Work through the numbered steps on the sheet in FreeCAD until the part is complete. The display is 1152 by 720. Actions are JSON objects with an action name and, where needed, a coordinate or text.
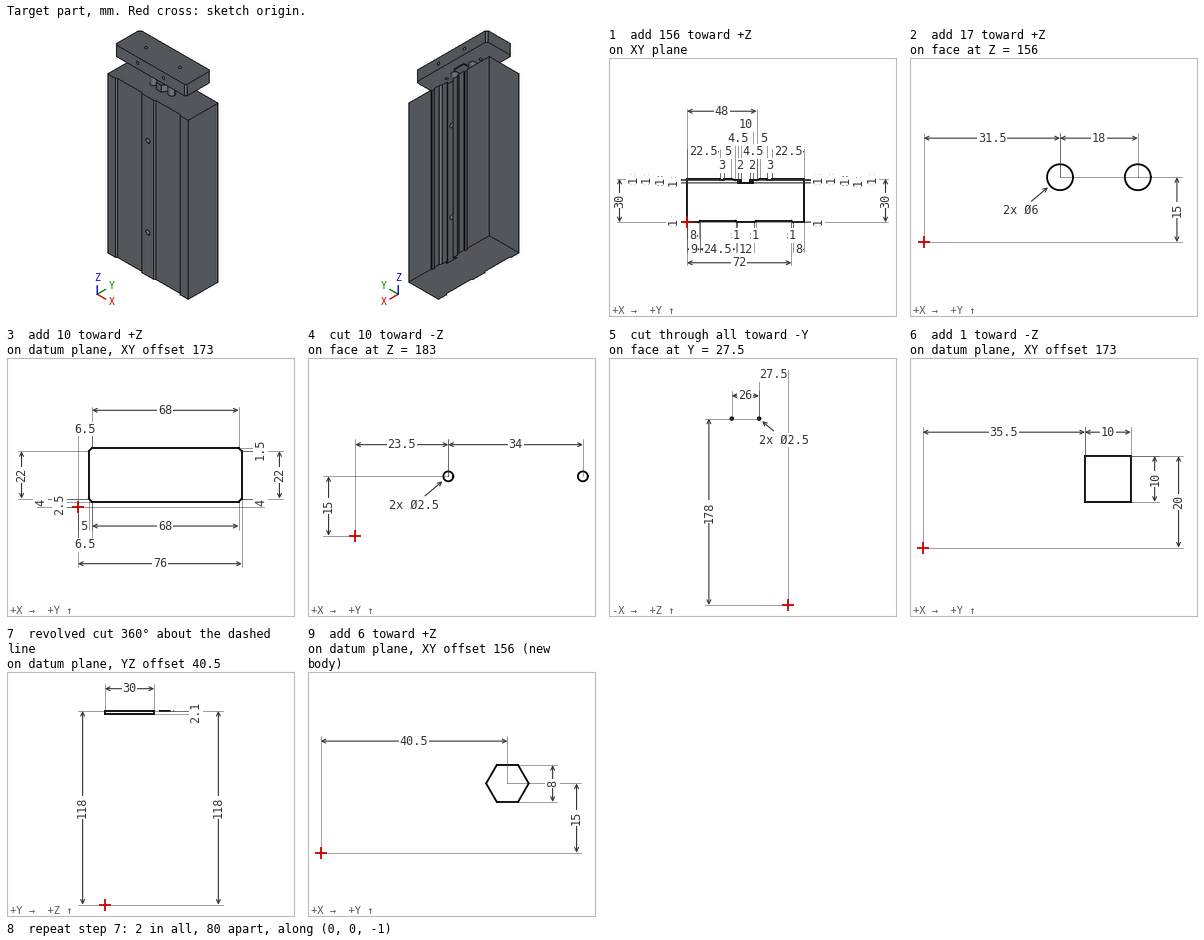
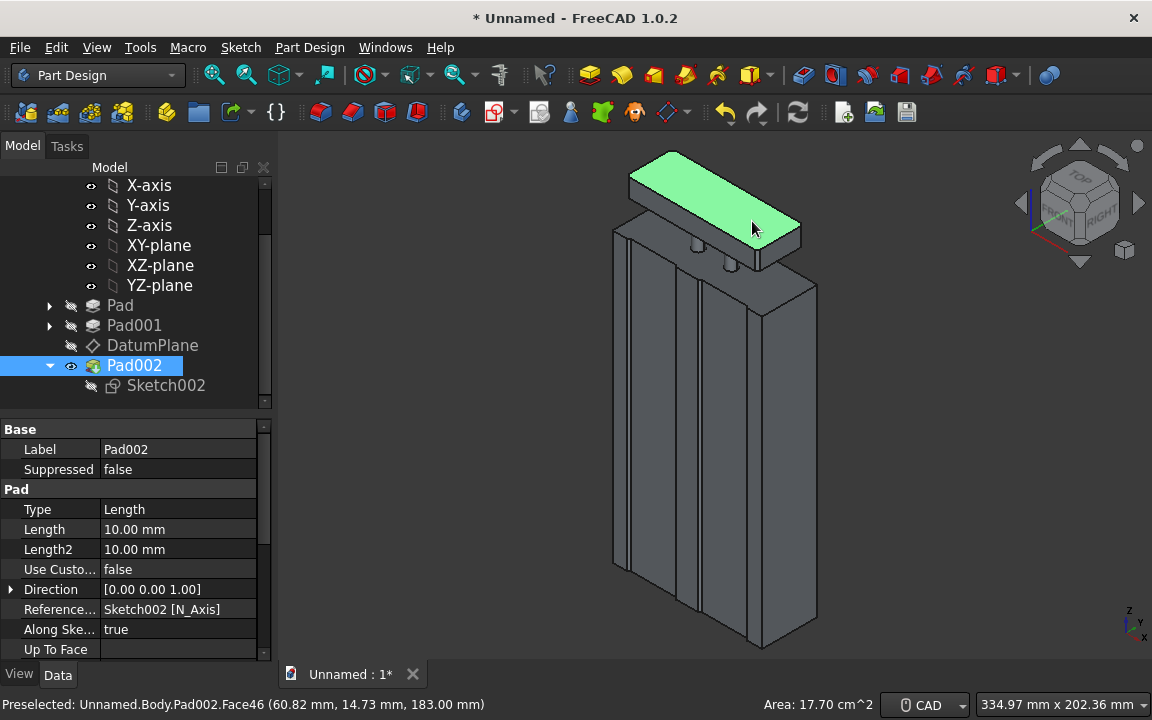
{"action": "left_click", "coordinate": [494, 112]}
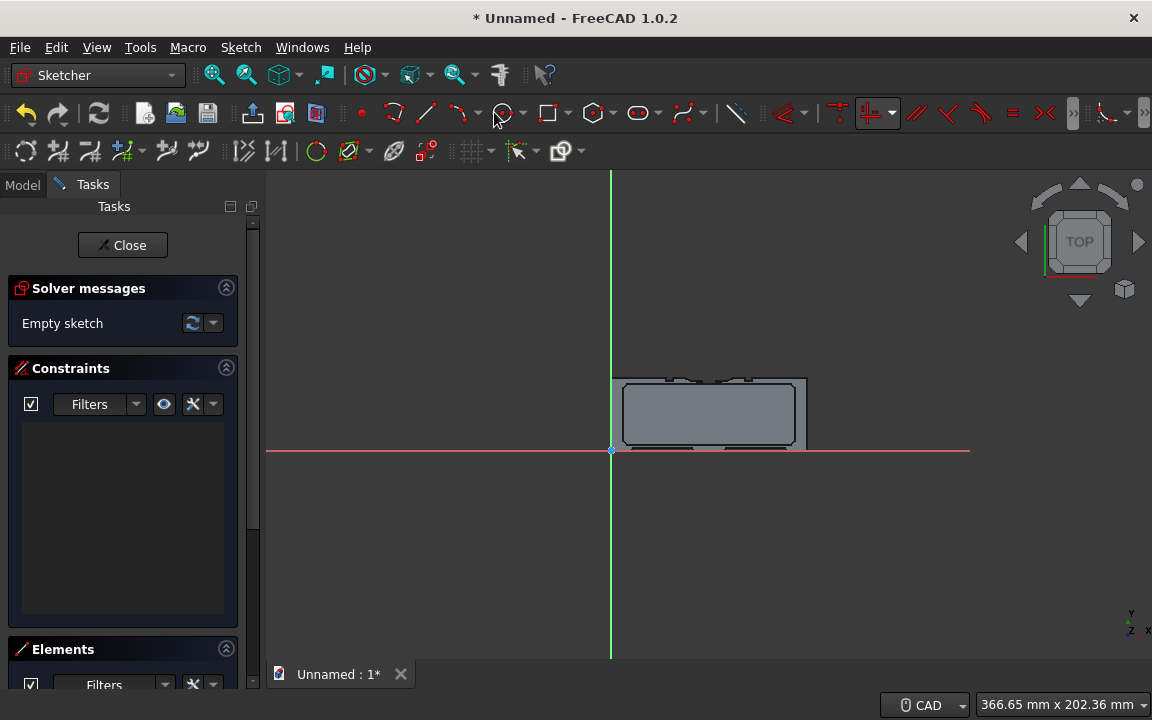
{"action": "scroll", "coordinate": [700, 438], "scroll_direction": "up", "scroll_amount": 6}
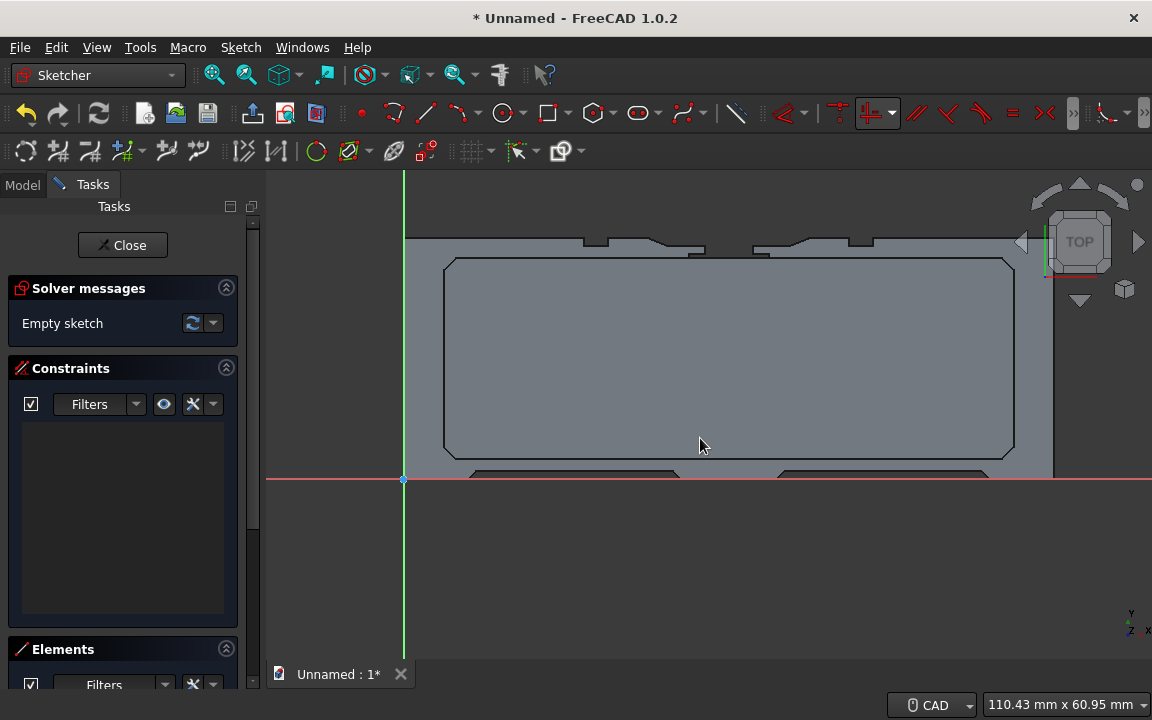
{"action": "left_click", "coordinate": [504, 114]}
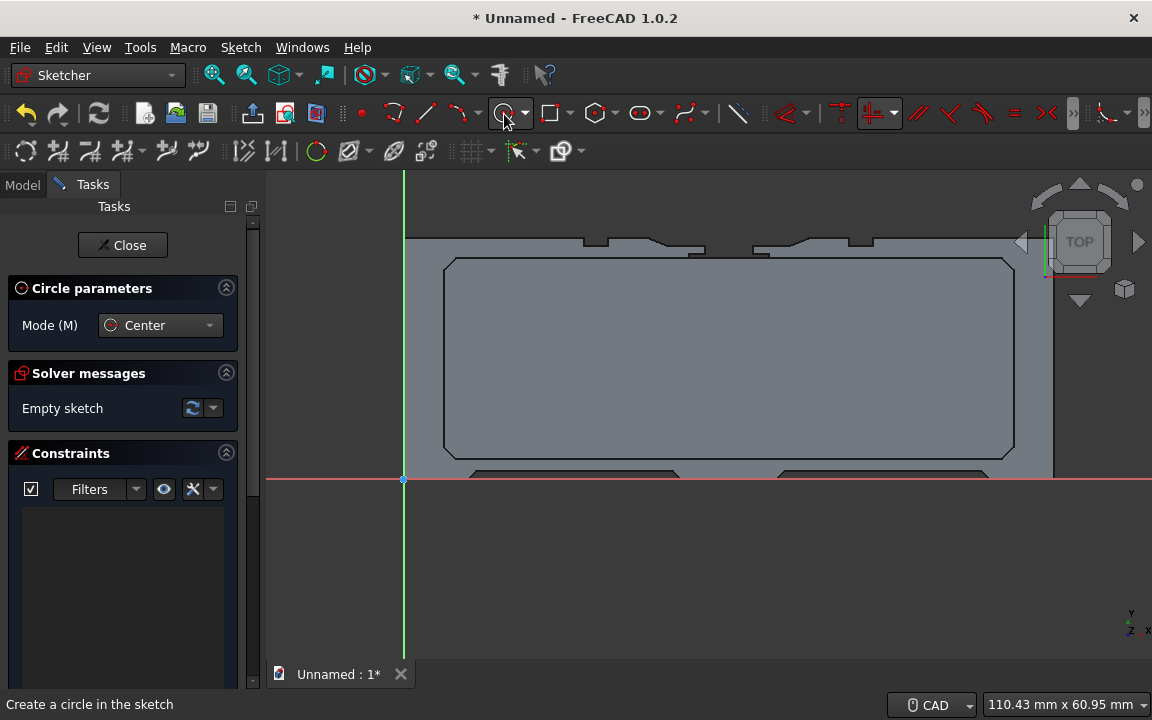
{"action": "scroll", "coordinate": [592, 359], "scroll_direction": "up", "scroll_amount": 5}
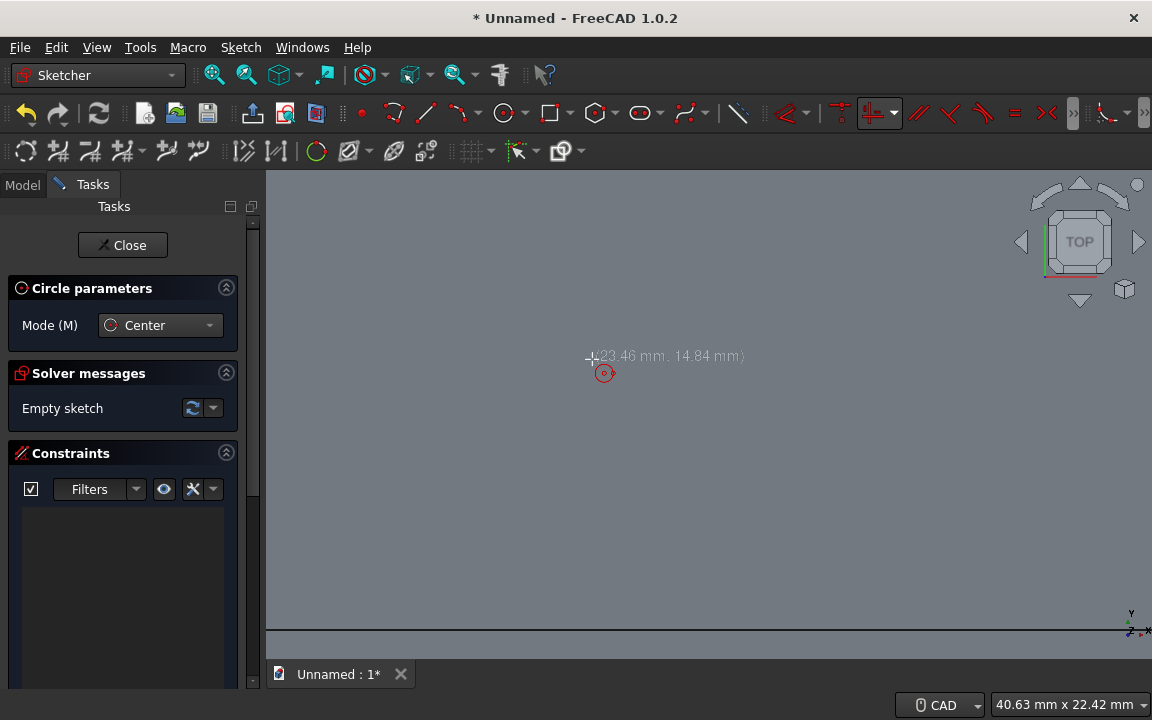
{"action": "left_click", "coordinate": [592, 358]}
{"action": "mouse_move", "coordinate": [612, 338]}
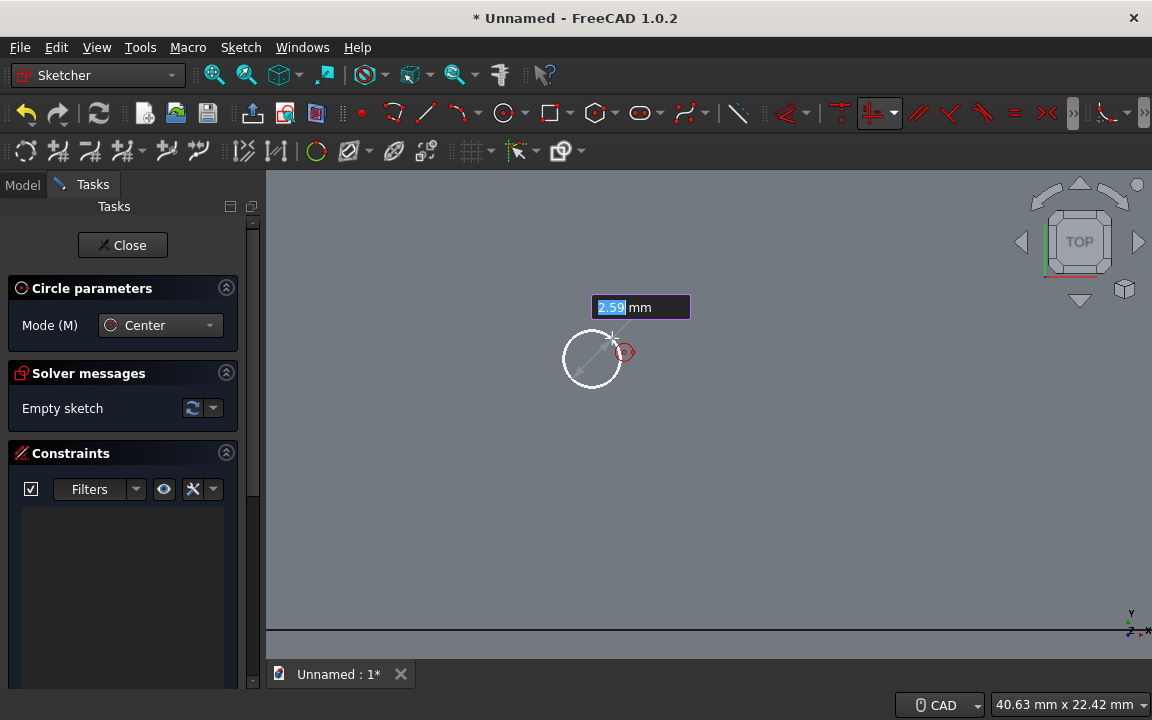
{"action": "type", "text": "2.5"}
{"action": "key", "text": "Return"}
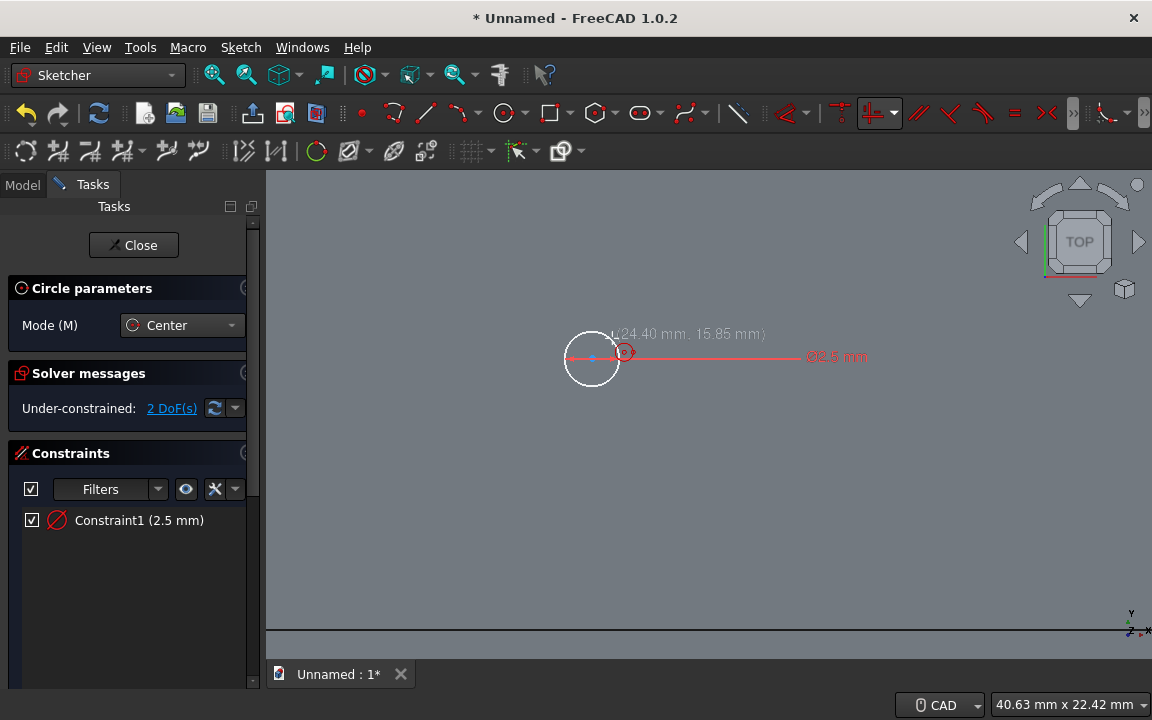
{"action": "scroll", "coordinate": [594, 360], "scroll_direction": "down", "scroll_amount": 5}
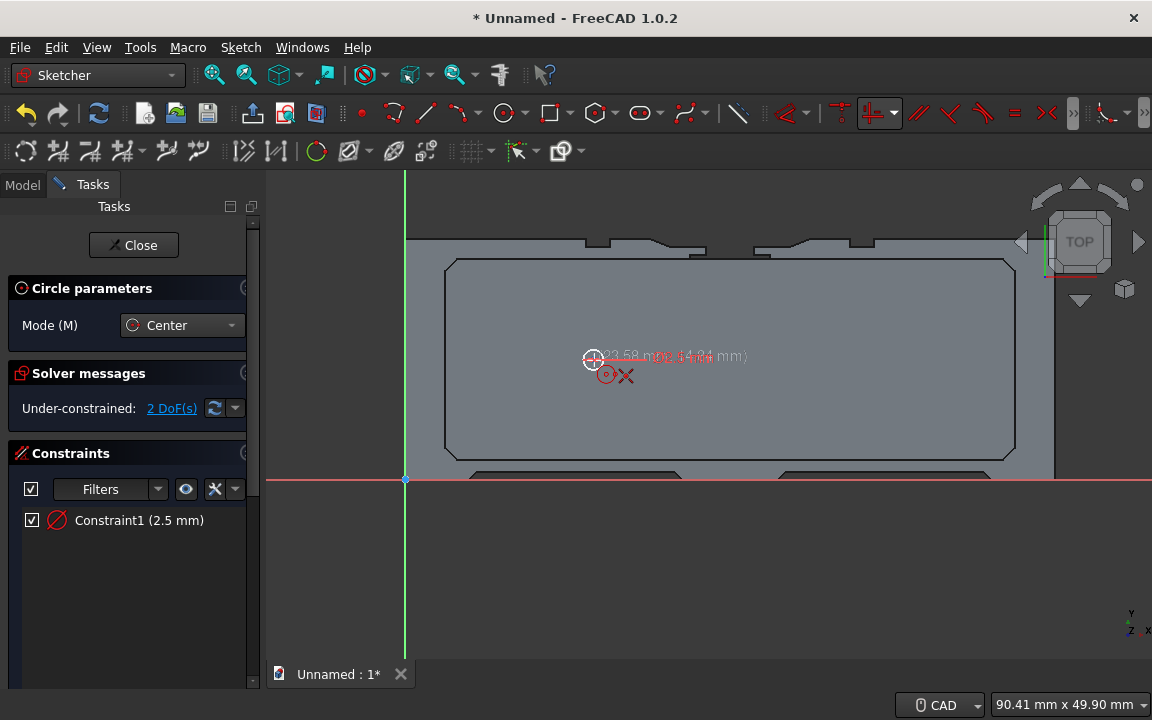
{"action": "scroll", "coordinate": [866, 359], "scroll_direction": "up", "scroll_amount": 5}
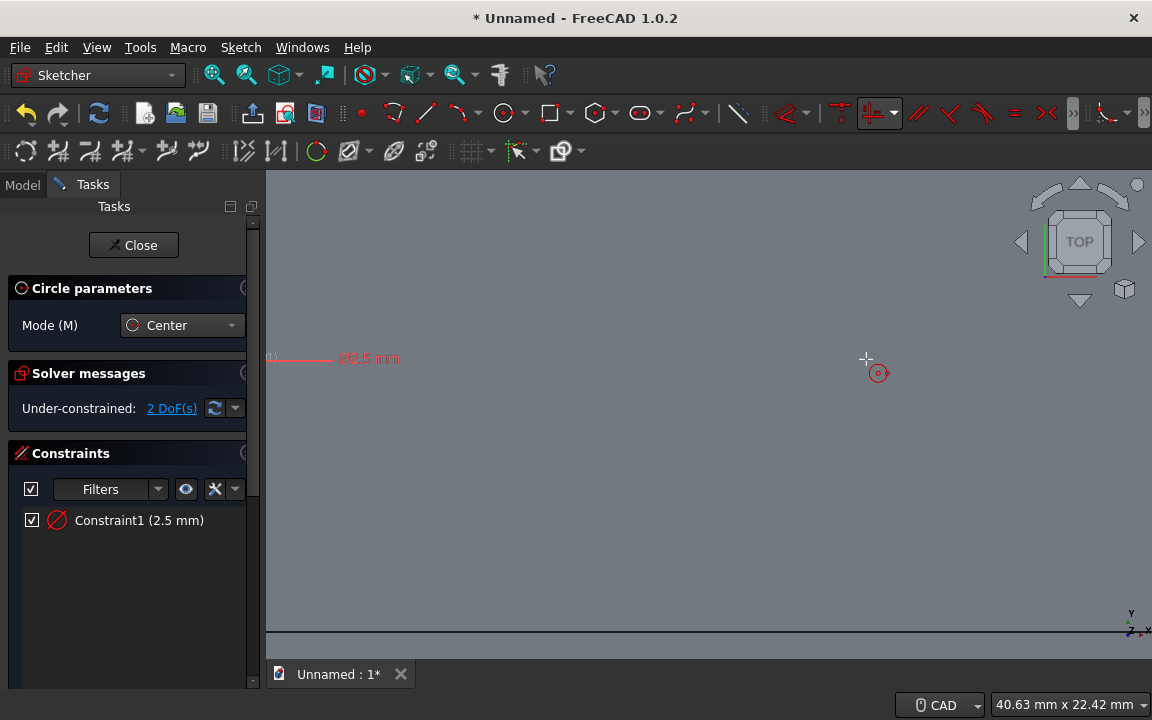
{"action": "left_click", "coordinate": [866, 359]}
{"action": "mouse_move", "coordinate": [885, 340]}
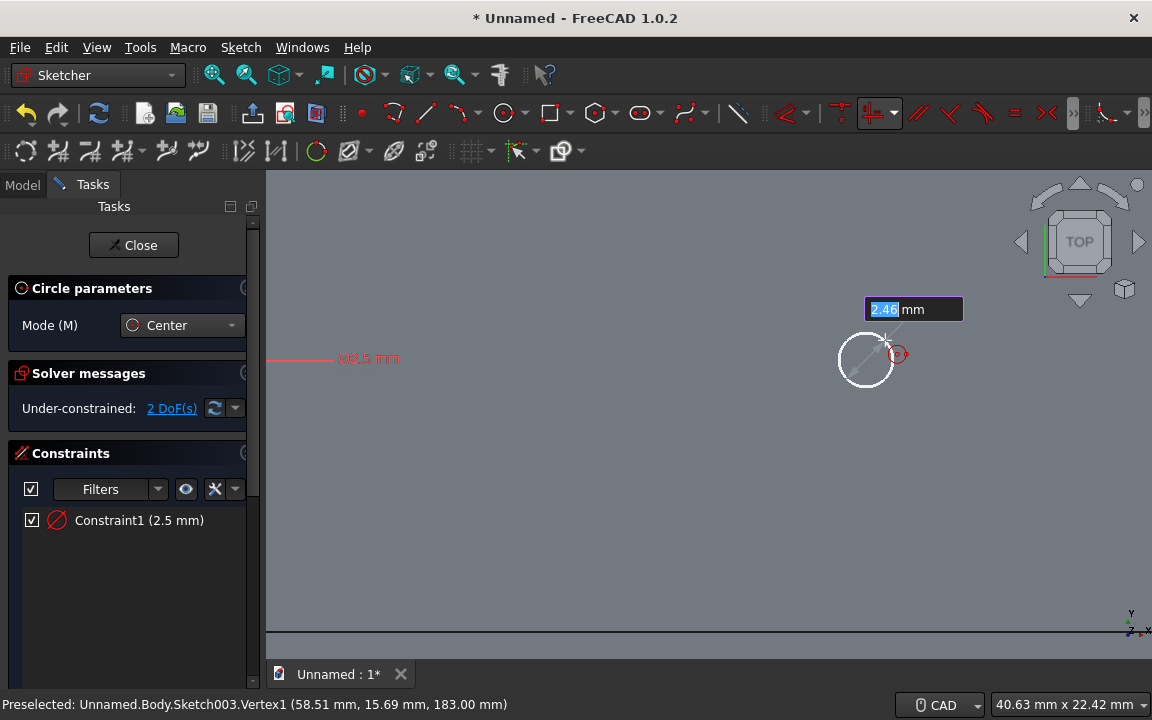
{"action": "type", "text": "2.5"}
{"action": "key", "text": "Return"}
{"action": "key", "text": "Escape"}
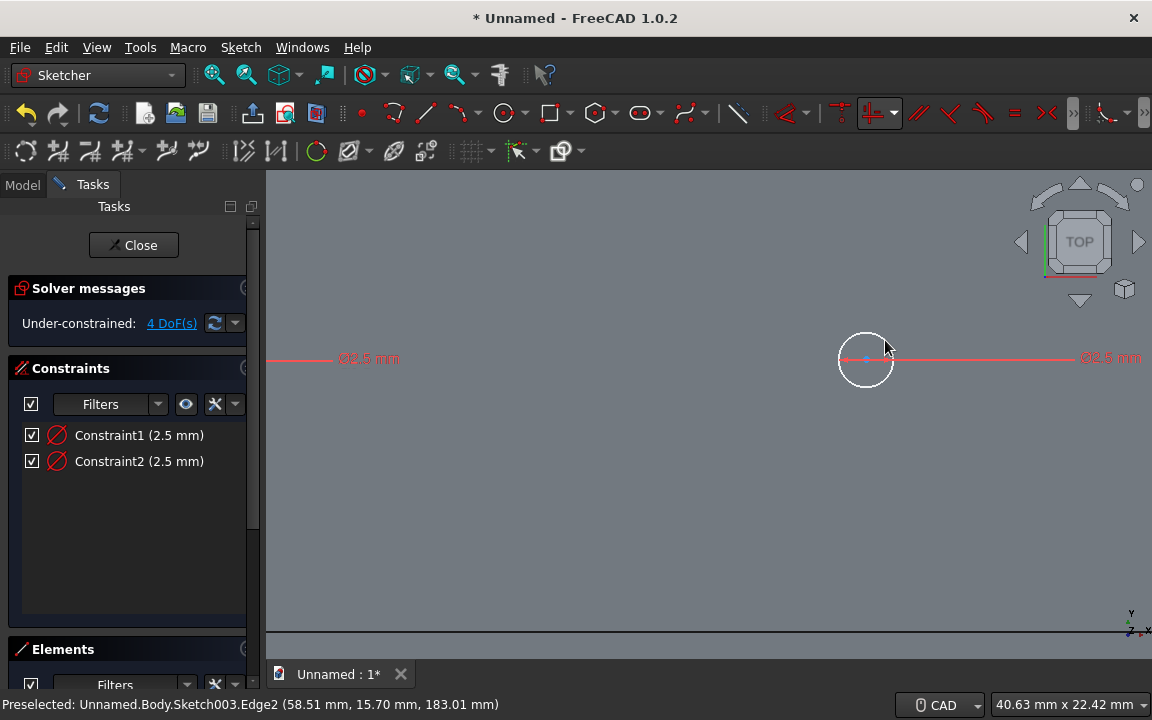
{"action": "scroll", "coordinate": [866, 359], "scroll_direction": "down", "scroll_amount": 5}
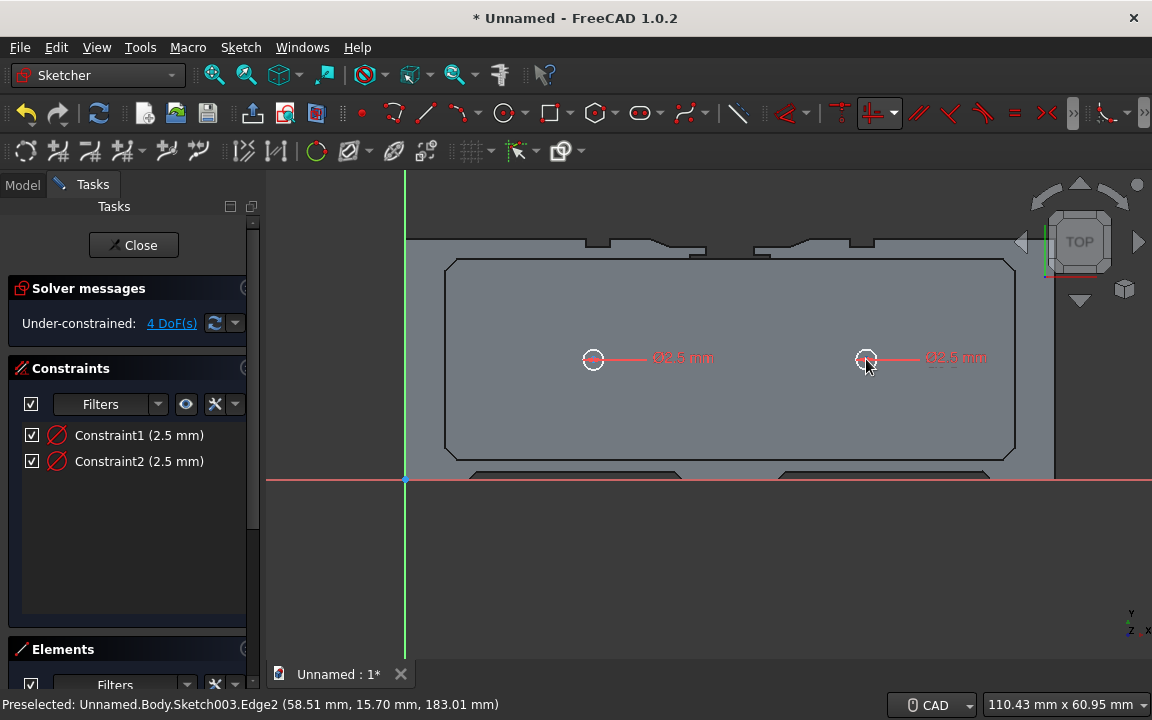
{"action": "left_click", "coordinate": [593, 360]}